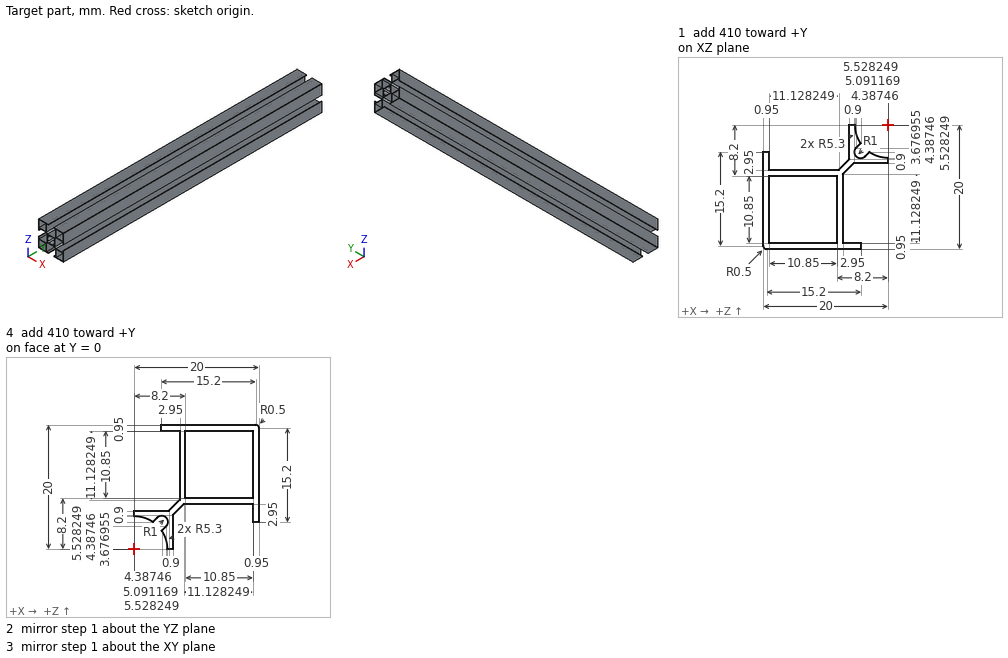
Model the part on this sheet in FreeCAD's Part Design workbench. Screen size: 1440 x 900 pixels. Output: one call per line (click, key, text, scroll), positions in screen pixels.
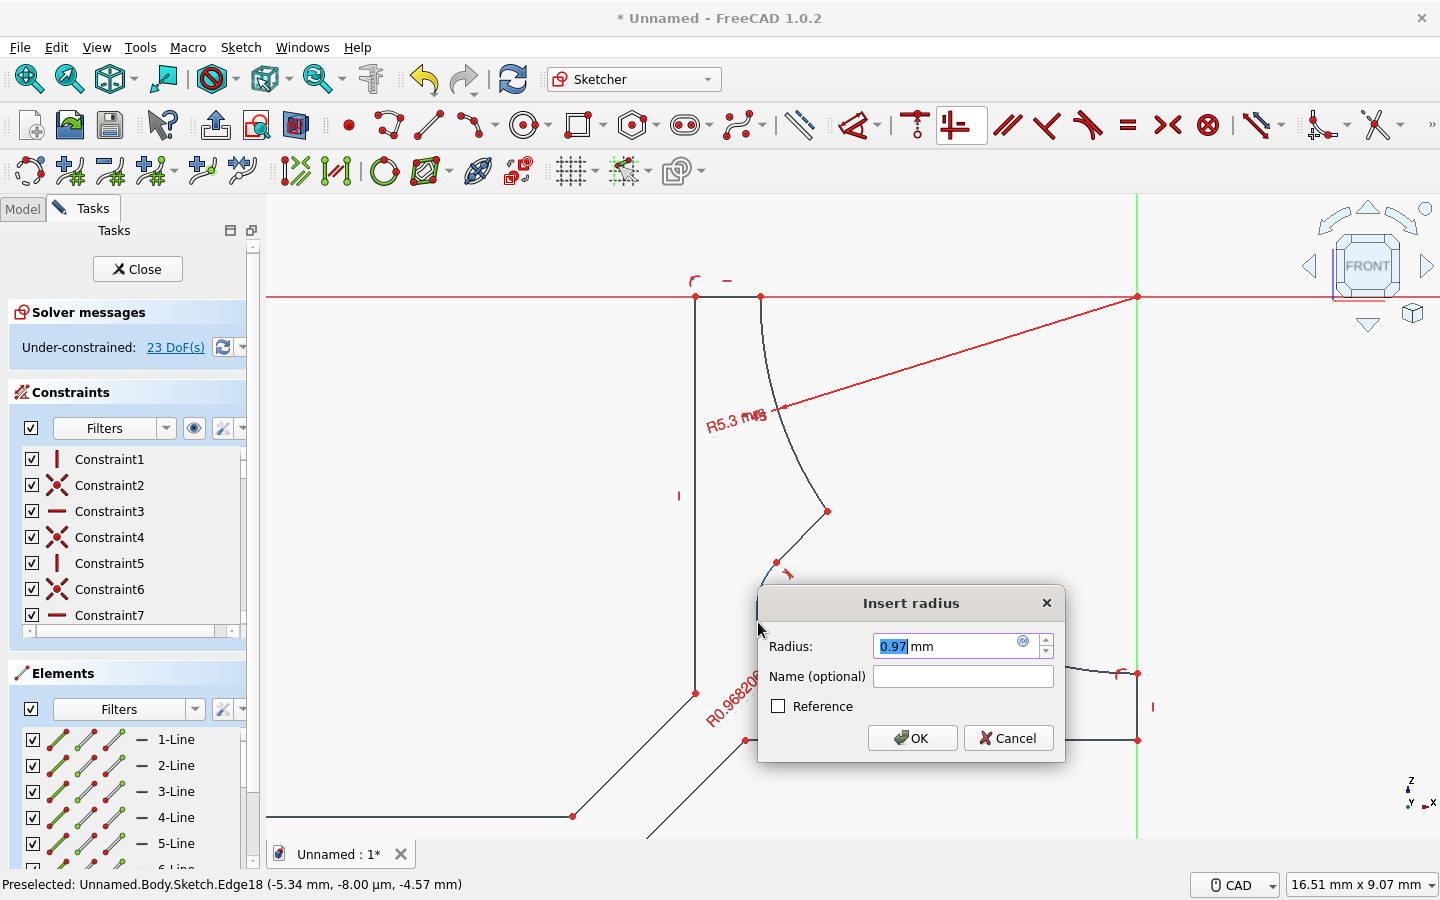
text(1)
key(Return)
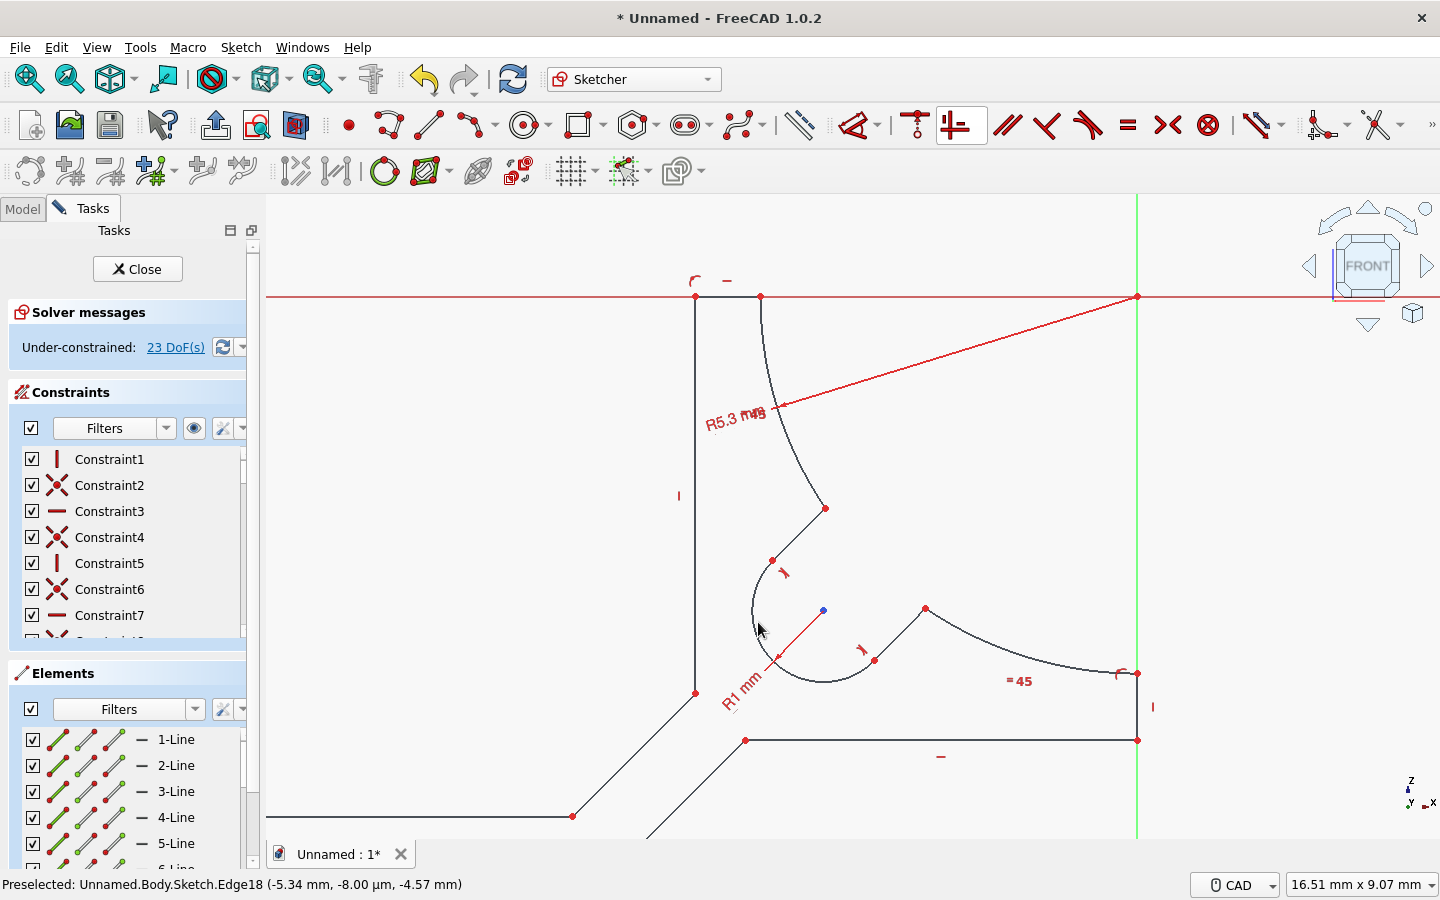
scroll(939, 305, down, 6)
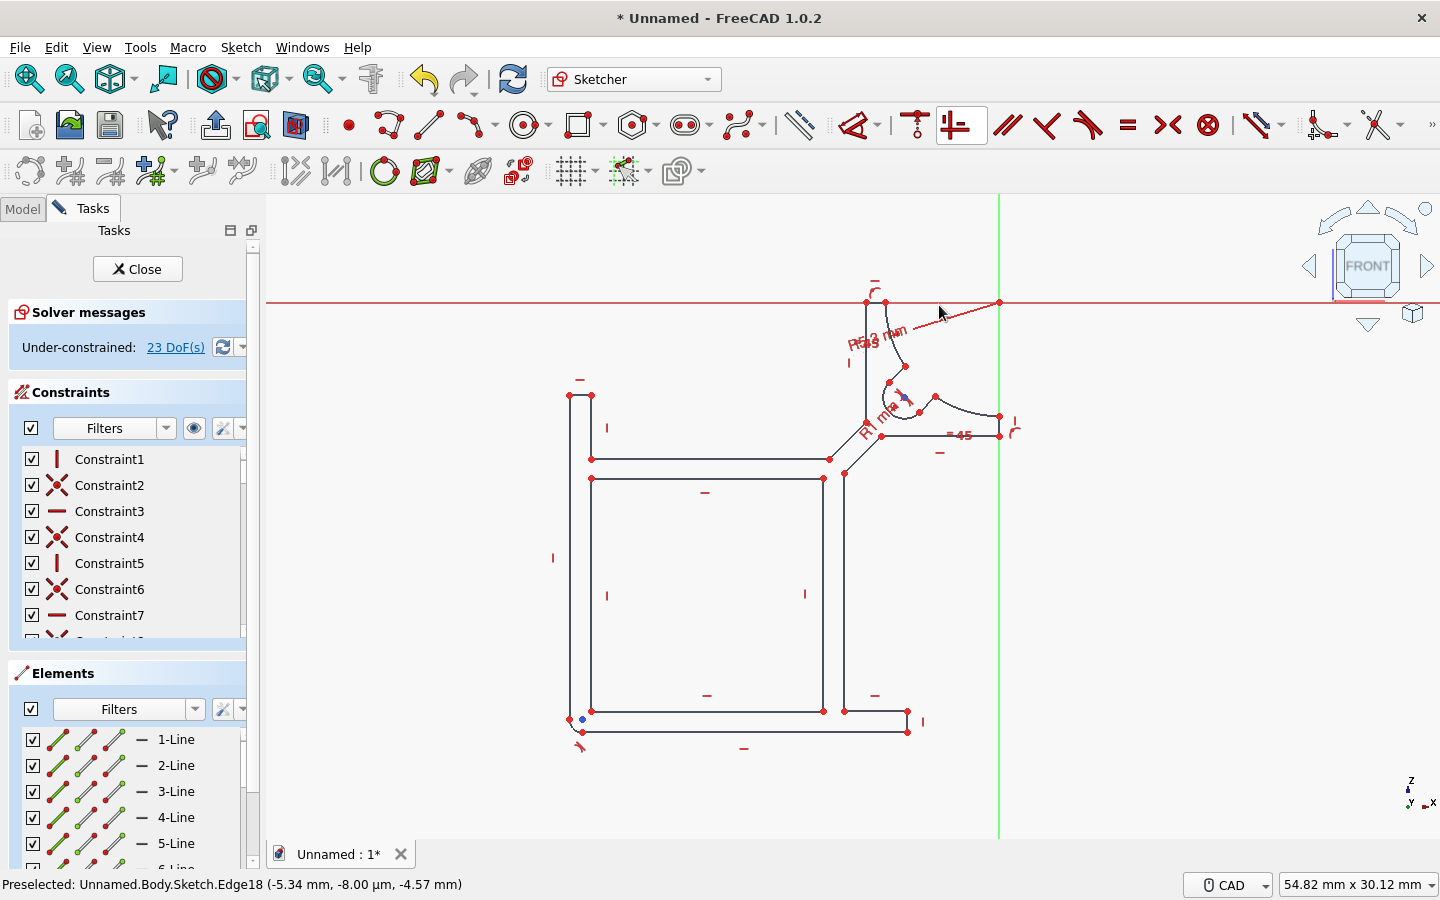
scroll(571, 726, up, 7)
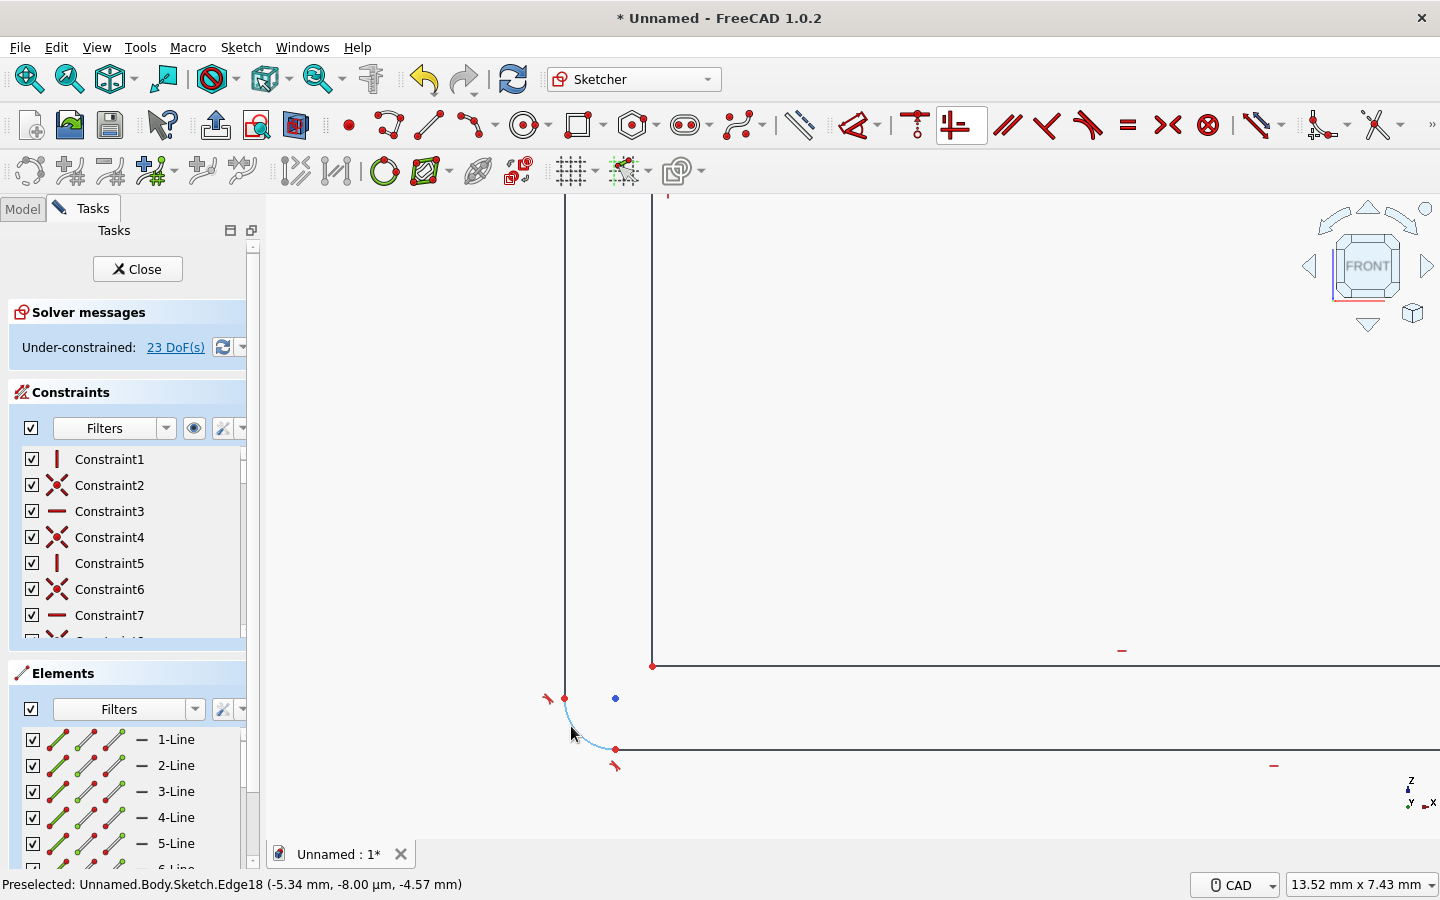
click(570, 722)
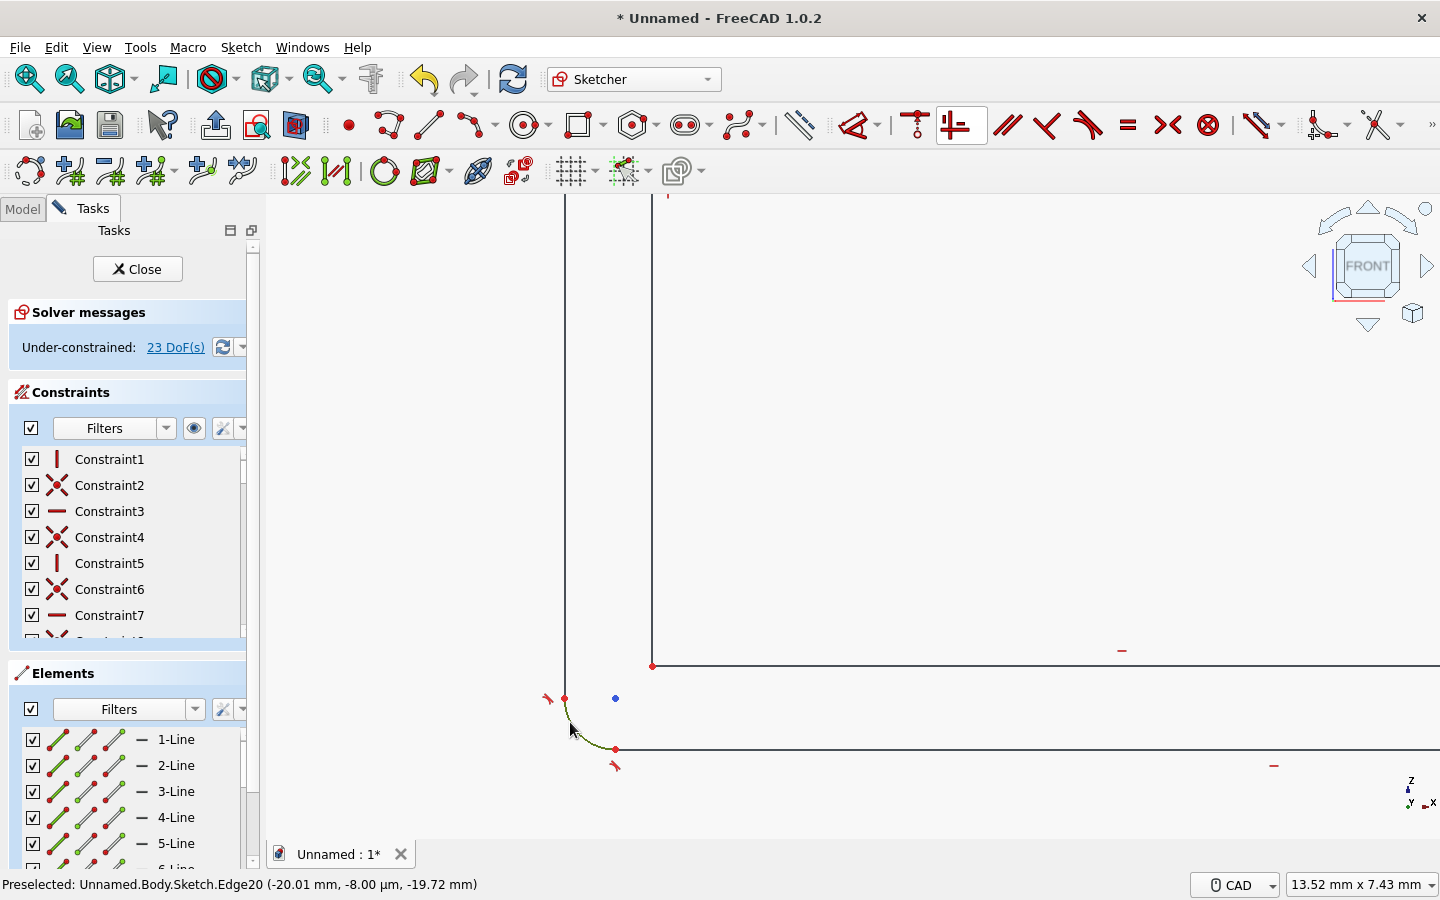
key(k)
key(r)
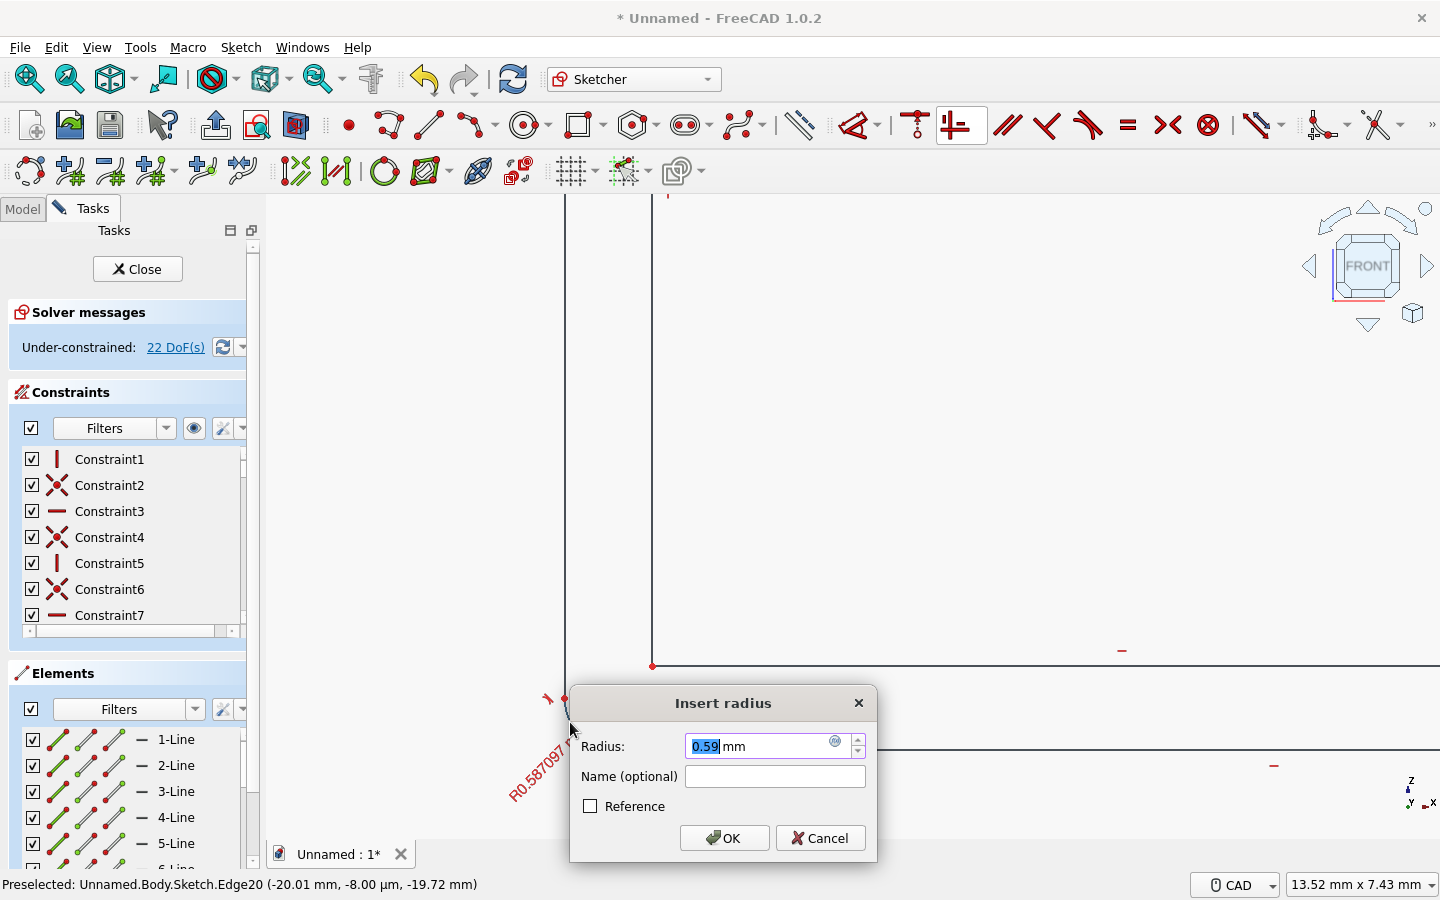
text(0.5)
key(Return)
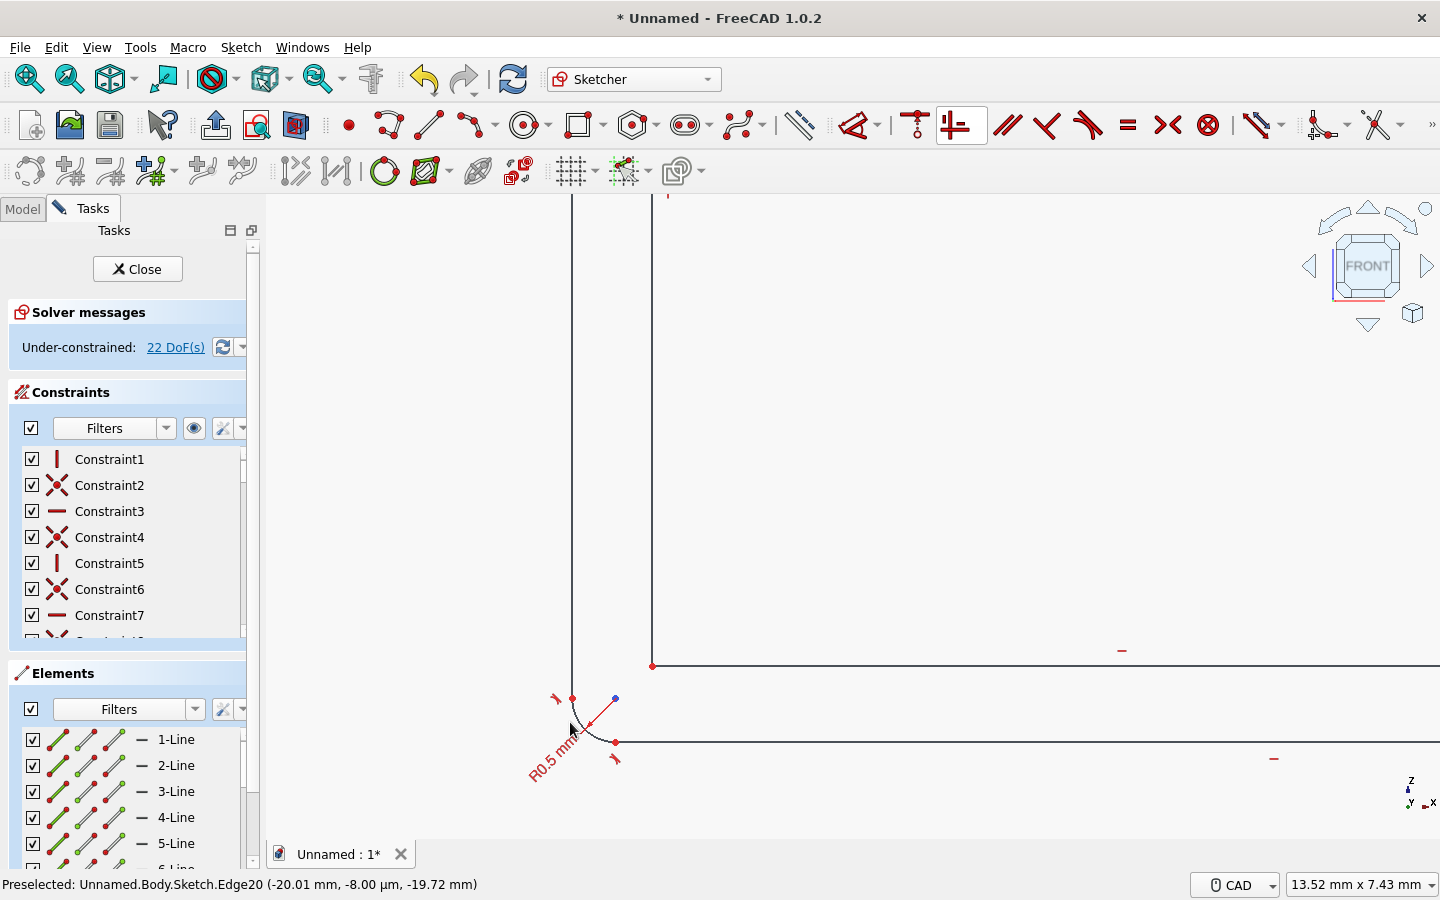
scroll(571, 726, down, 7)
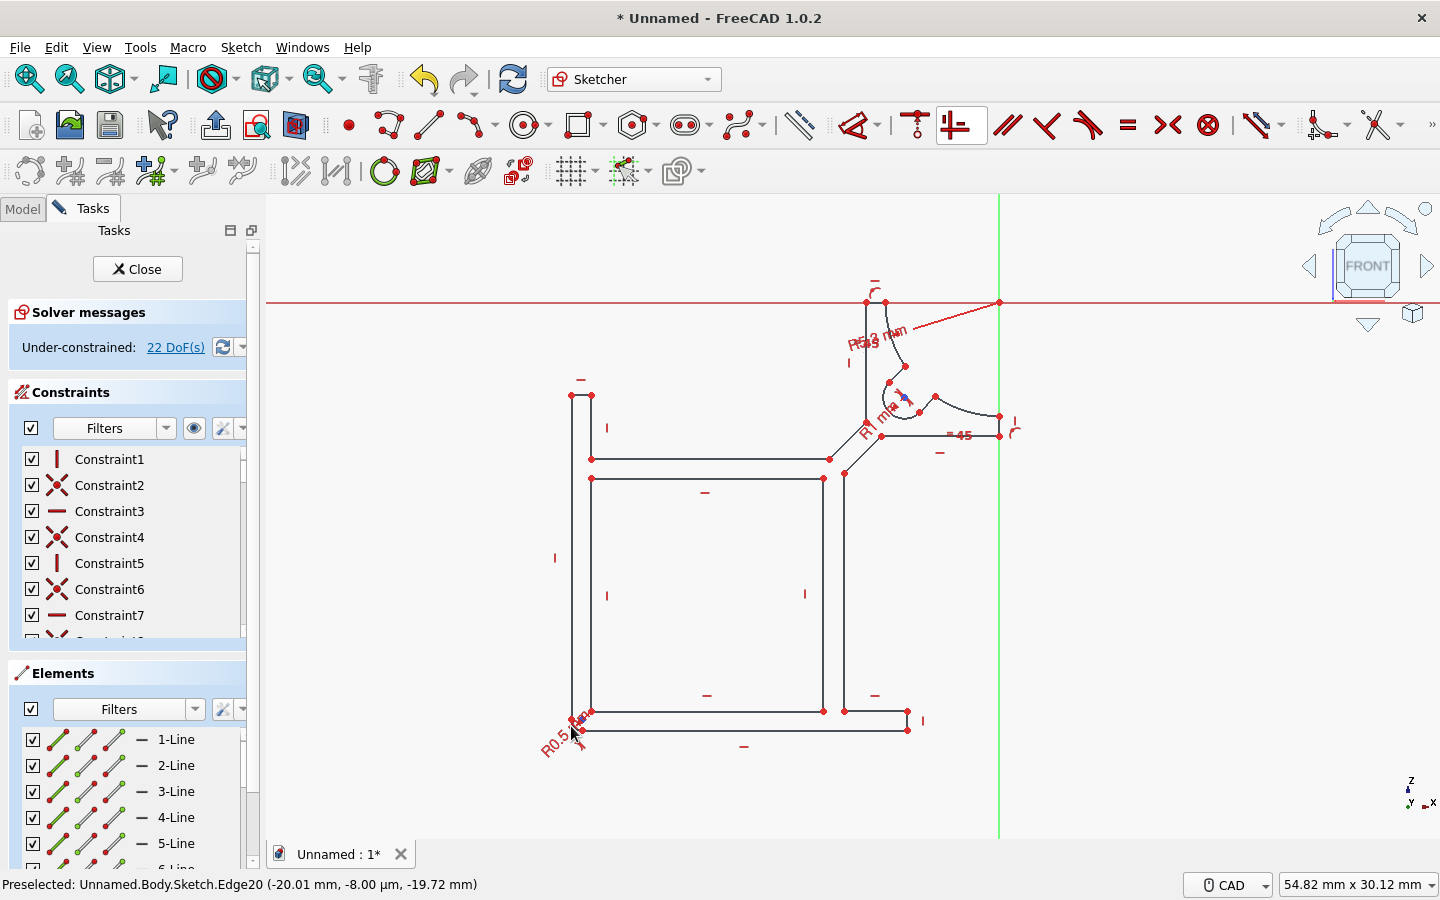
scroll(872, 303, up, 5)